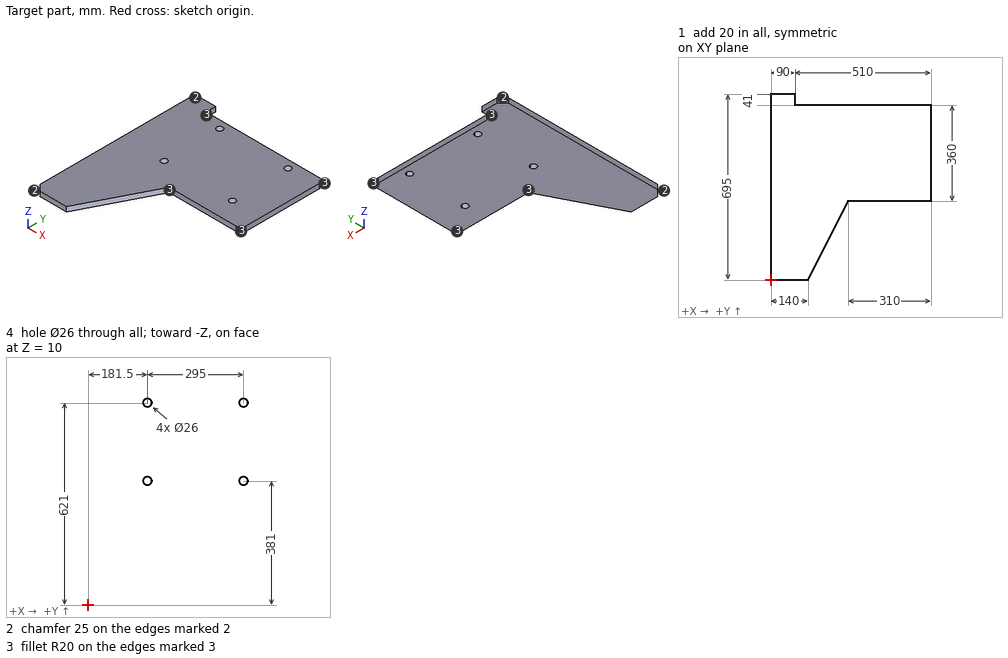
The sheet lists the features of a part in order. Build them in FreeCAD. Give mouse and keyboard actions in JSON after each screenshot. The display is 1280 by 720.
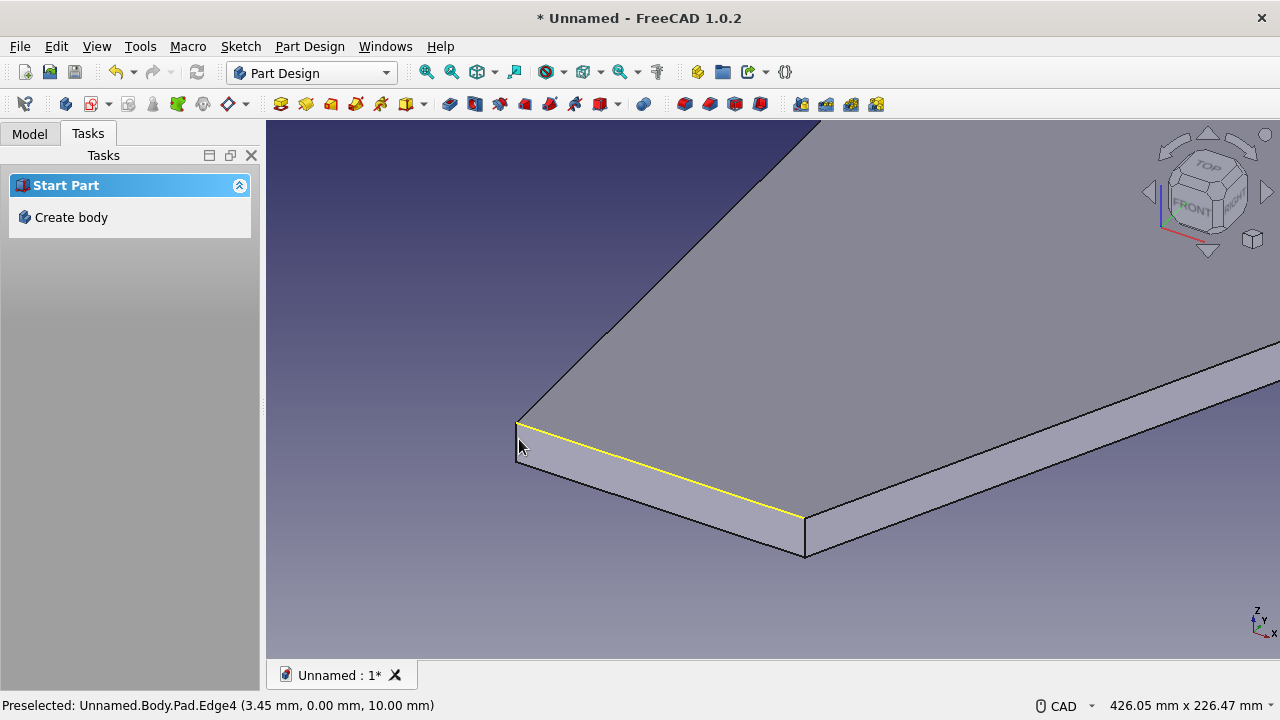
{"action": "left_click", "coordinate": [427, 72]}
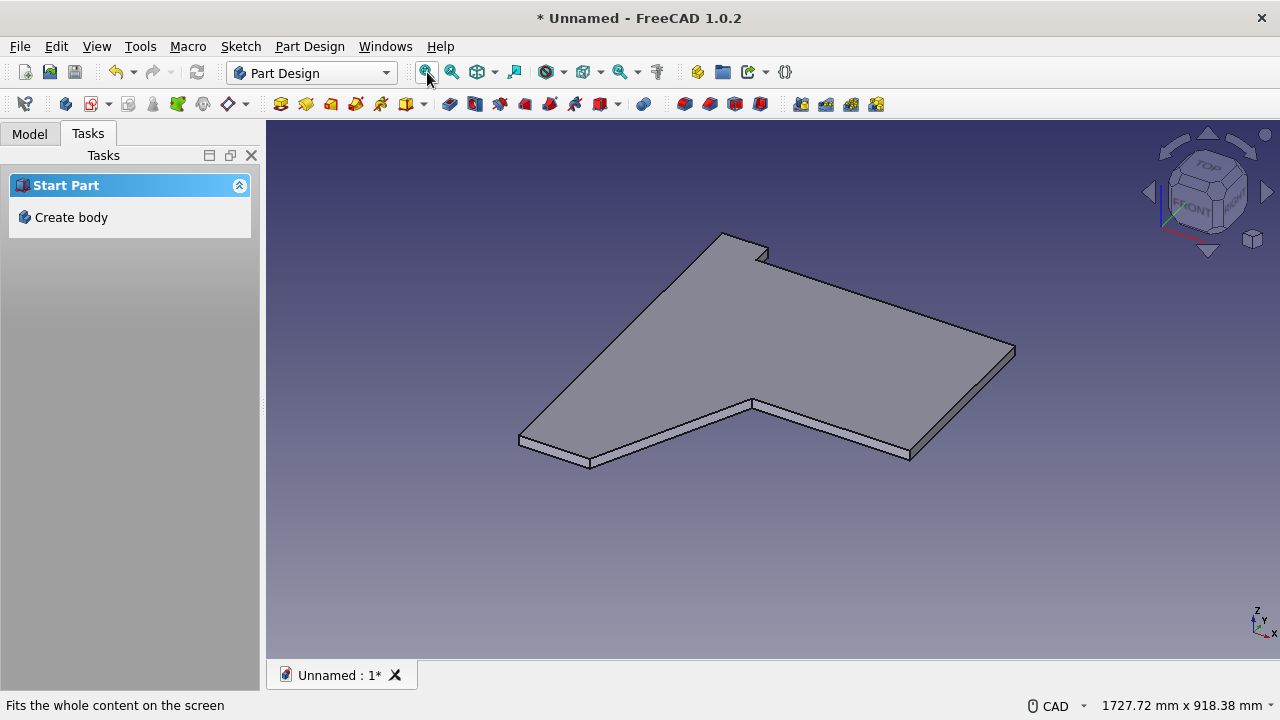
{"action": "key", "text": "0"}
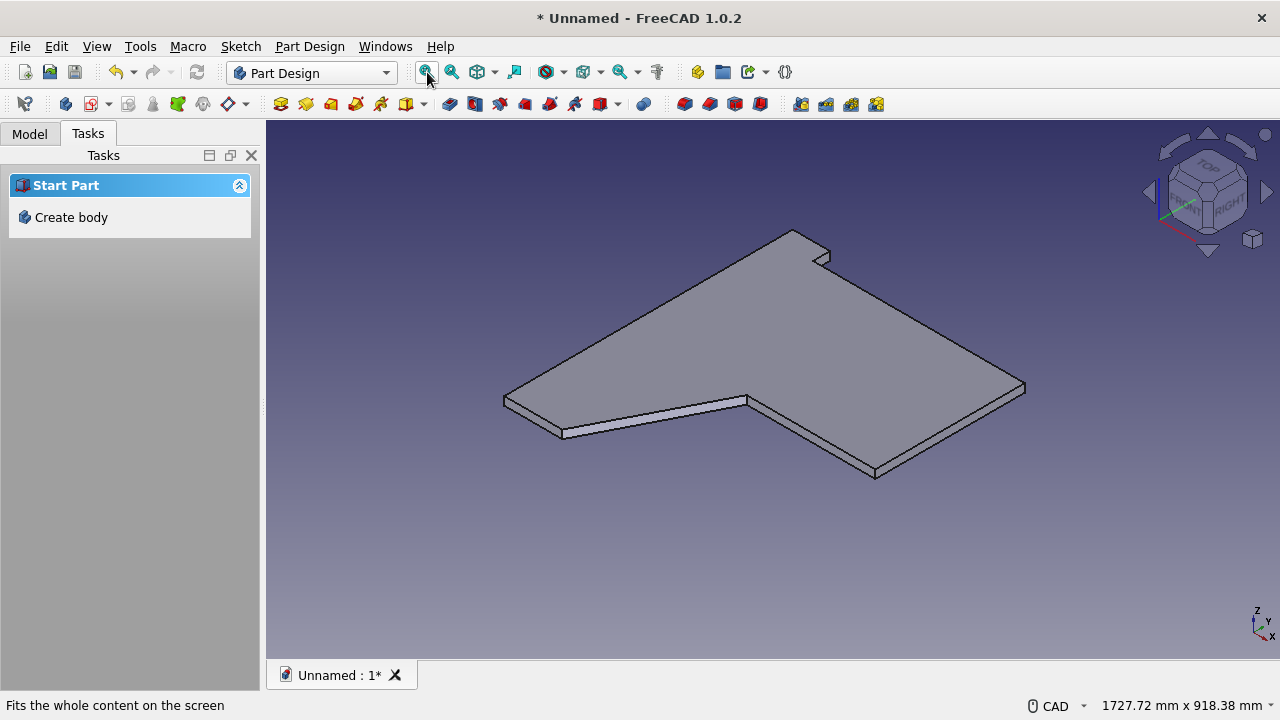
{"action": "scroll", "coordinate": [504, 400], "scroll_direction": "up", "scroll_amount": 7}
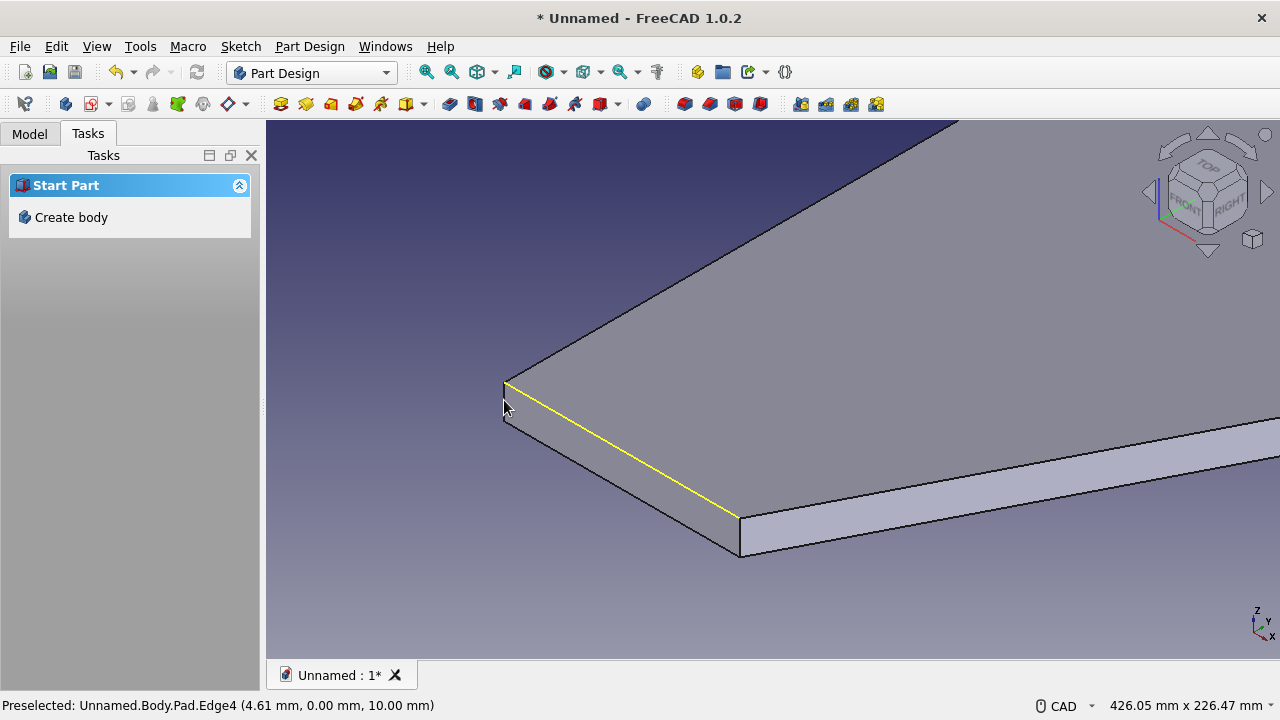
{"action": "left_click", "coordinate": [427, 72]}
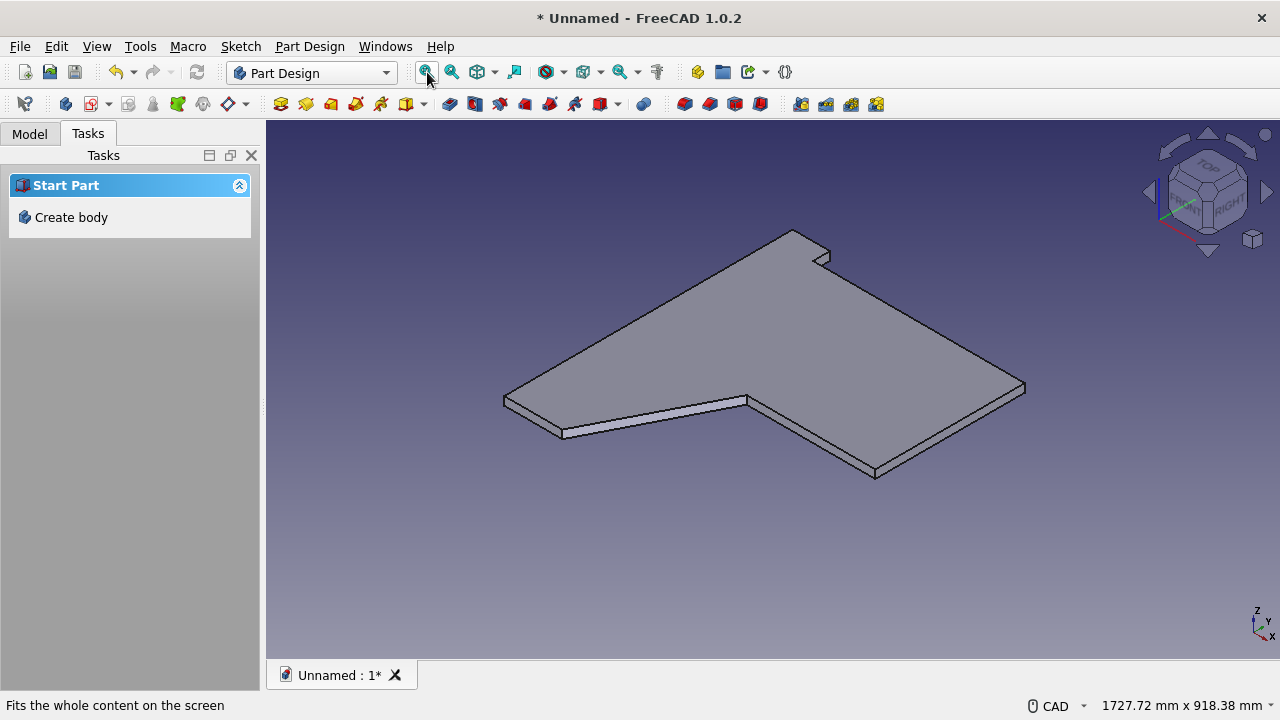
{"action": "key", "text": "2"}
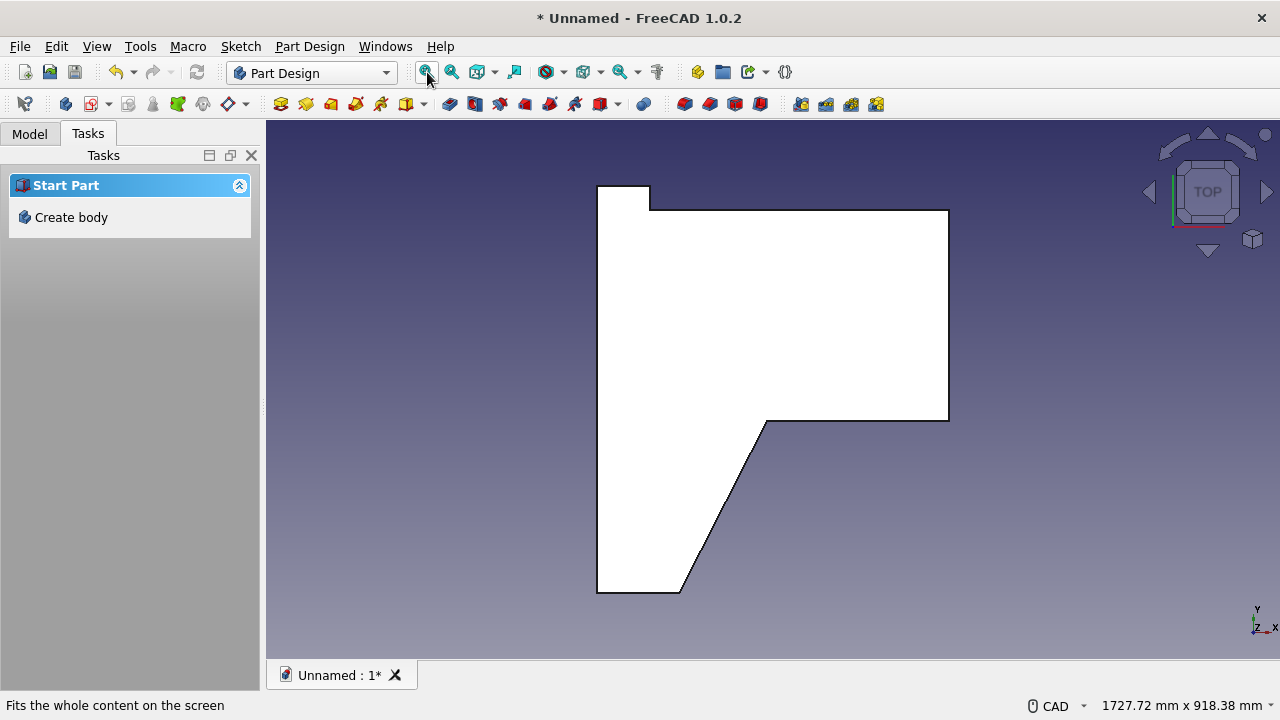
{"action": "scroll", "coordinate": [597, 592], "scroll_direction": "up", "scroll_amount": 7}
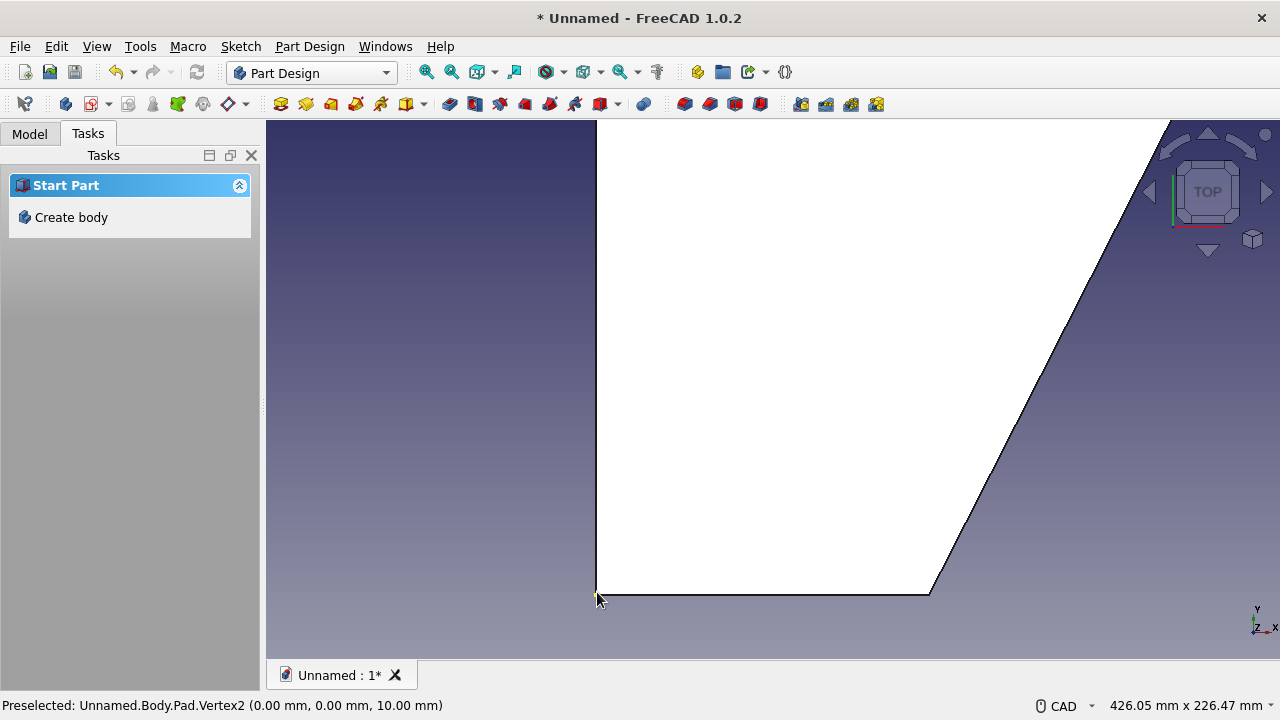
{"action": "left_click", "coordinate": [427, 72]}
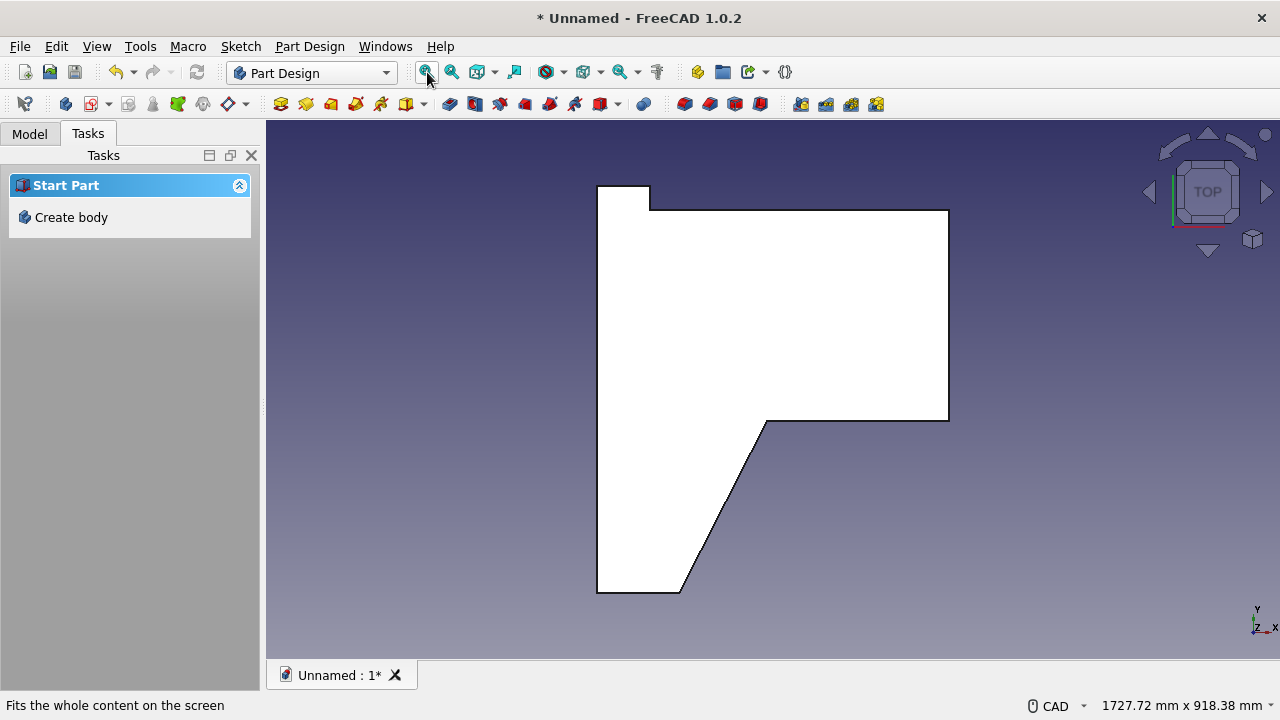
{"action": "key", "text": "1"}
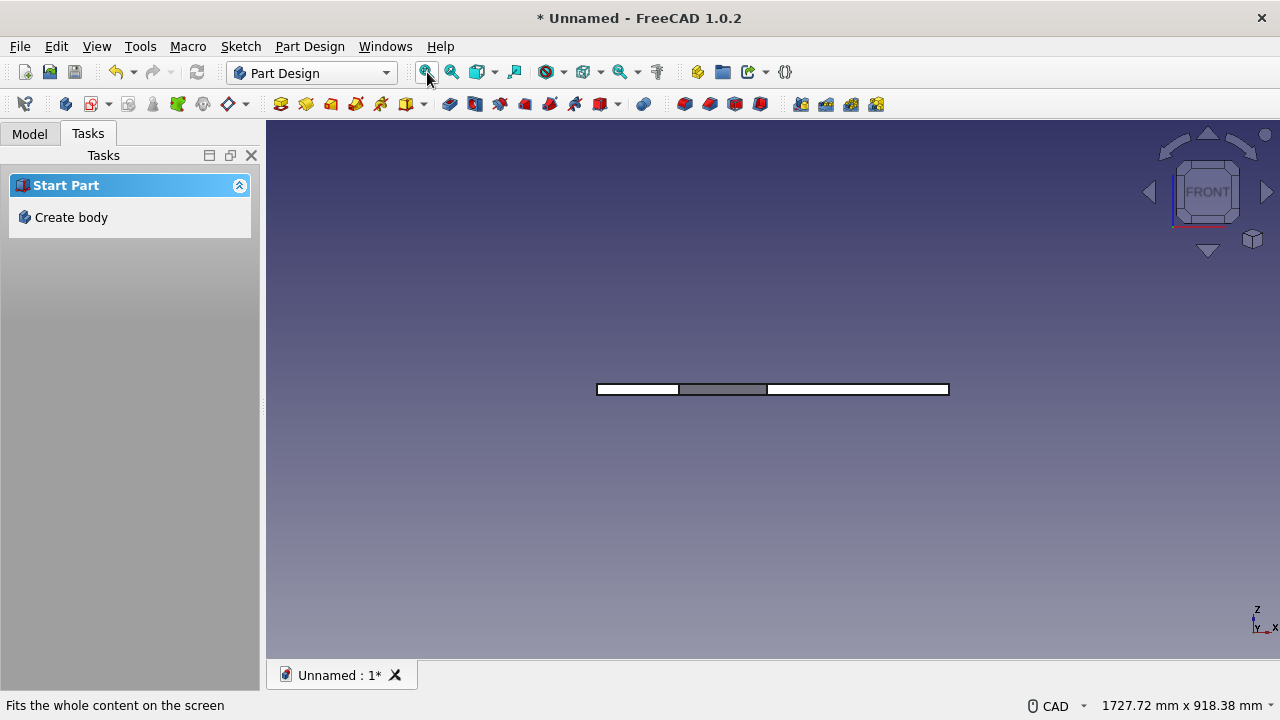
{"action": "left_click", "coordinate": [427, 72]}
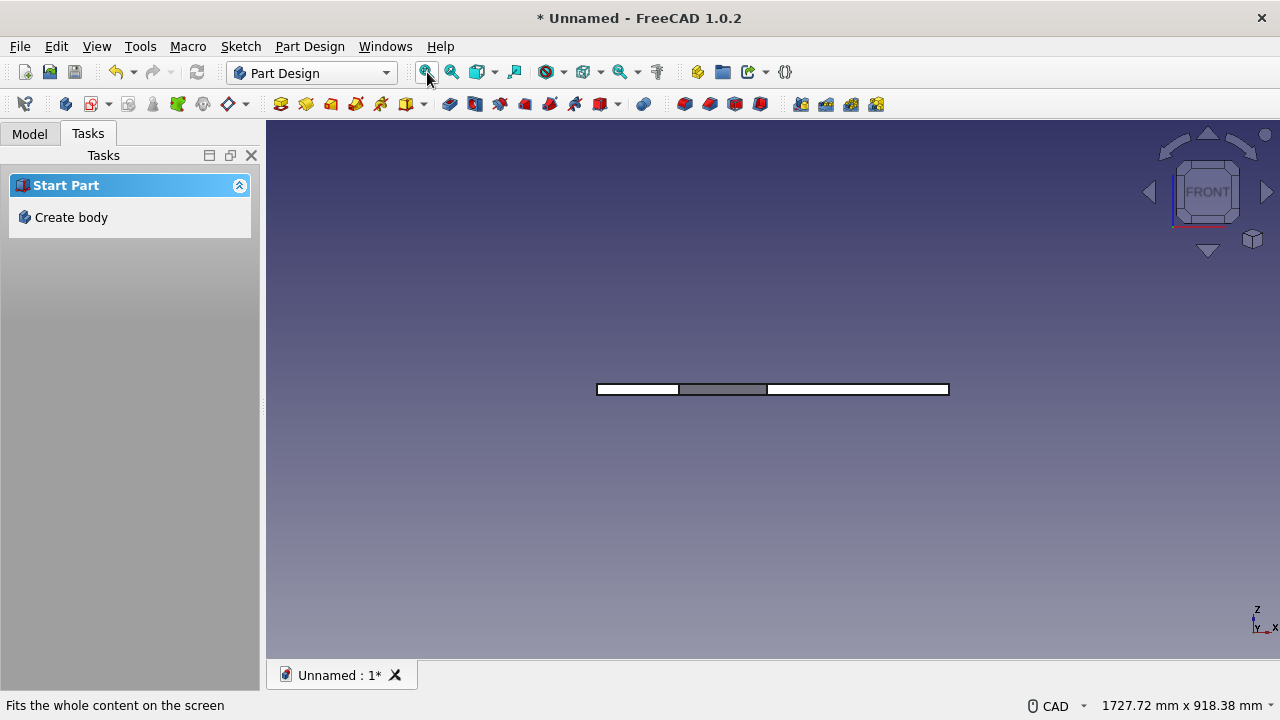
{"action": "scroll", "coordinate": [597, 389], "scroll_direction": "up", "scroll_amount": 7}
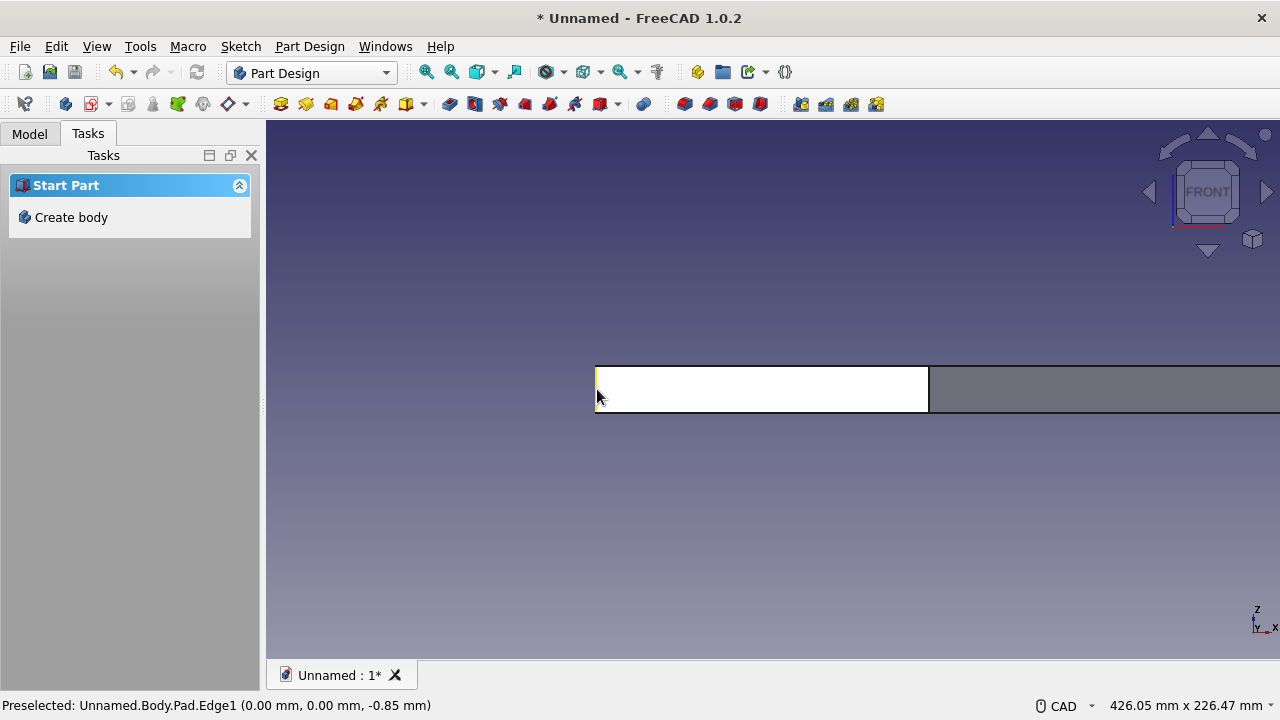
{"action": "left_click", "coordinate": [596, 389]}